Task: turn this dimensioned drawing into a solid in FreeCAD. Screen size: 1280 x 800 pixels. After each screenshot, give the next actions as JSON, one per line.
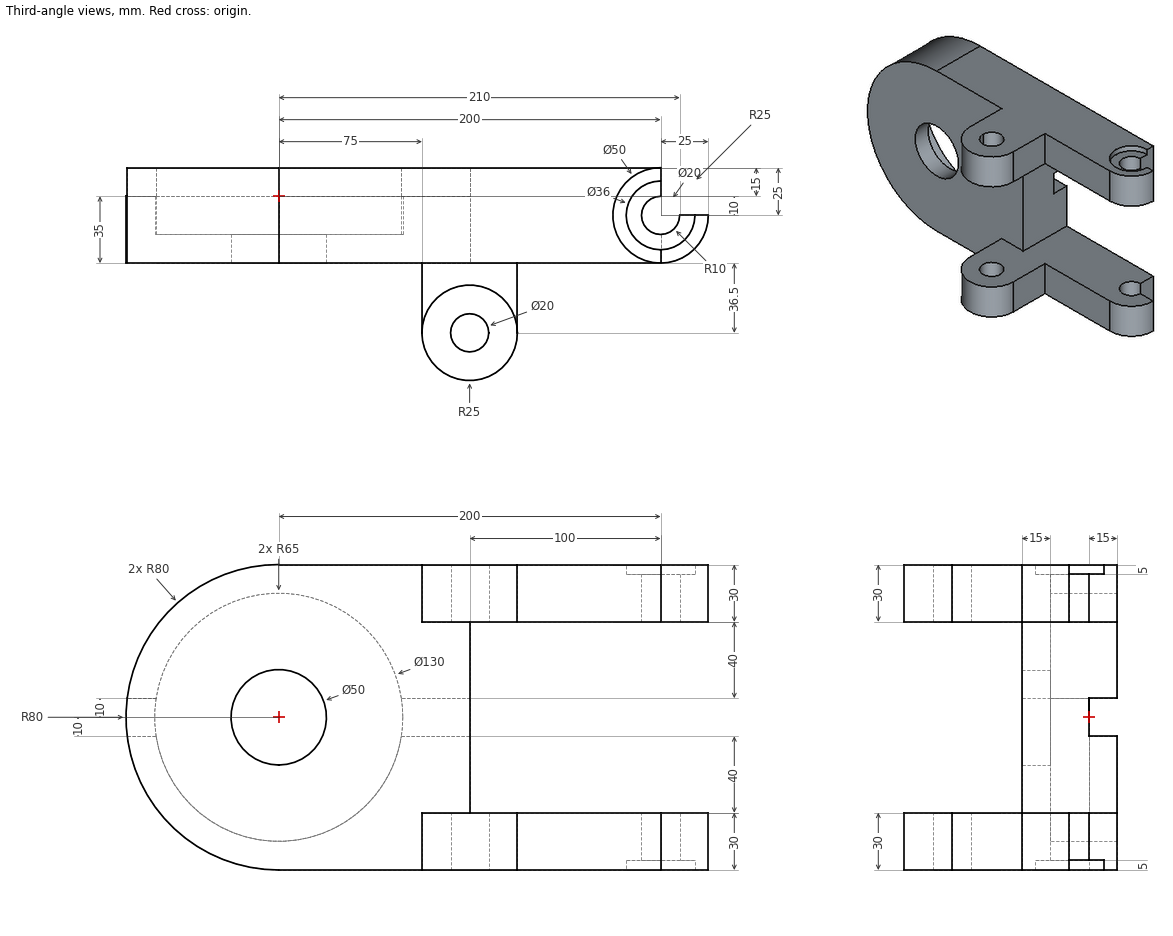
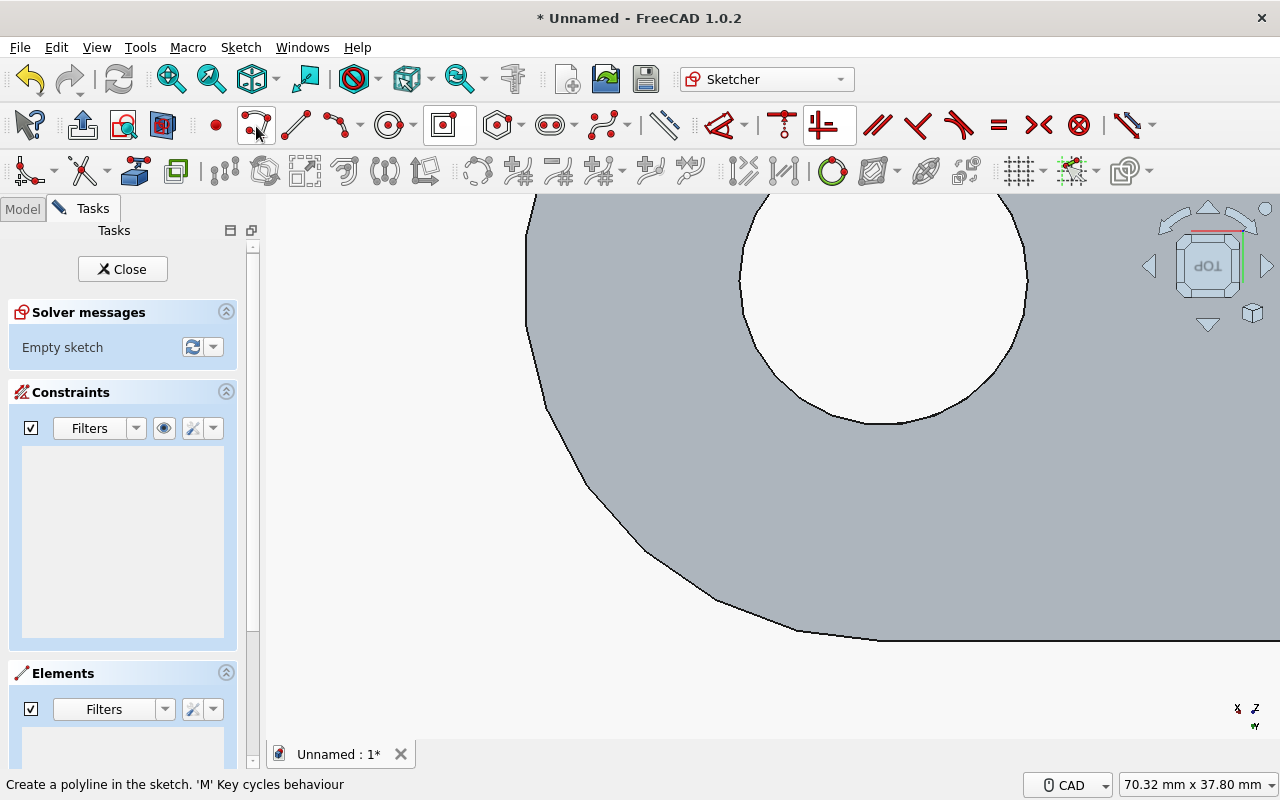
{"action": "left_click", "coordinate": [884, 641]}
{"action": "left_click", "coordinate": [884, 281]}
{"action": "left_click", "coordinate": [523, 281]}
{"action": "right_click", "coordinate": [523, 281]}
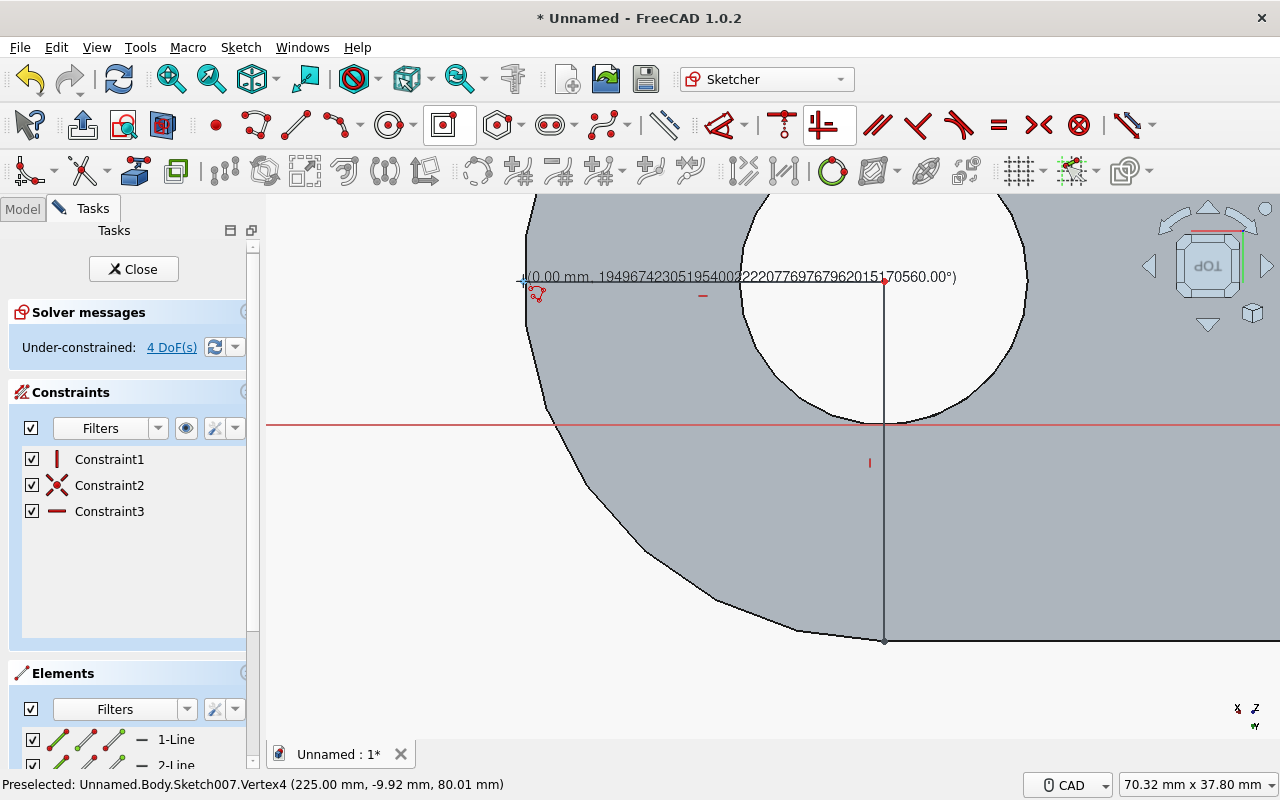
{"action": "left_click", "coordinate": [336, 126]}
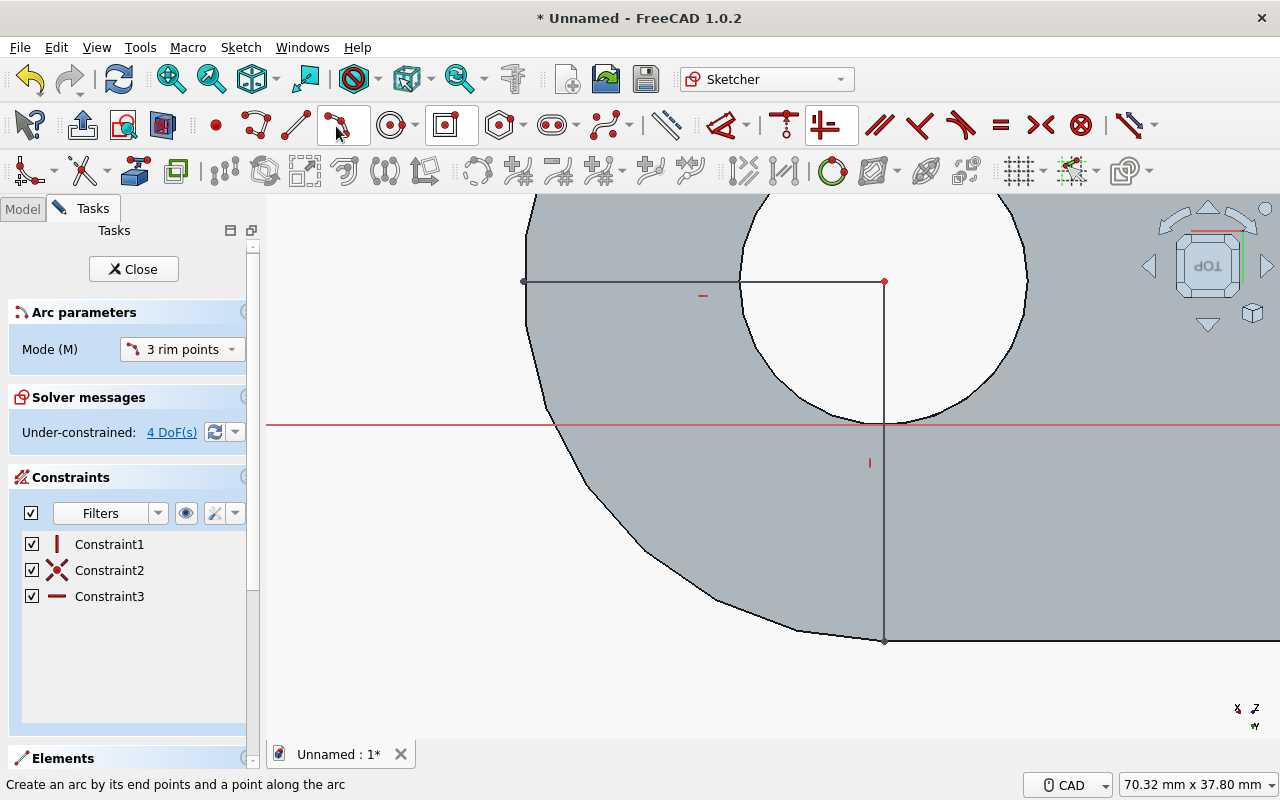
{"action": "left_click", "coordinate": [523, 282]}
{"action": "left_click", "coordinate": [884, 642]}
{"action": "left_click", "coordinate": [629, 536]}
{"action": "key", "text": "Escape"}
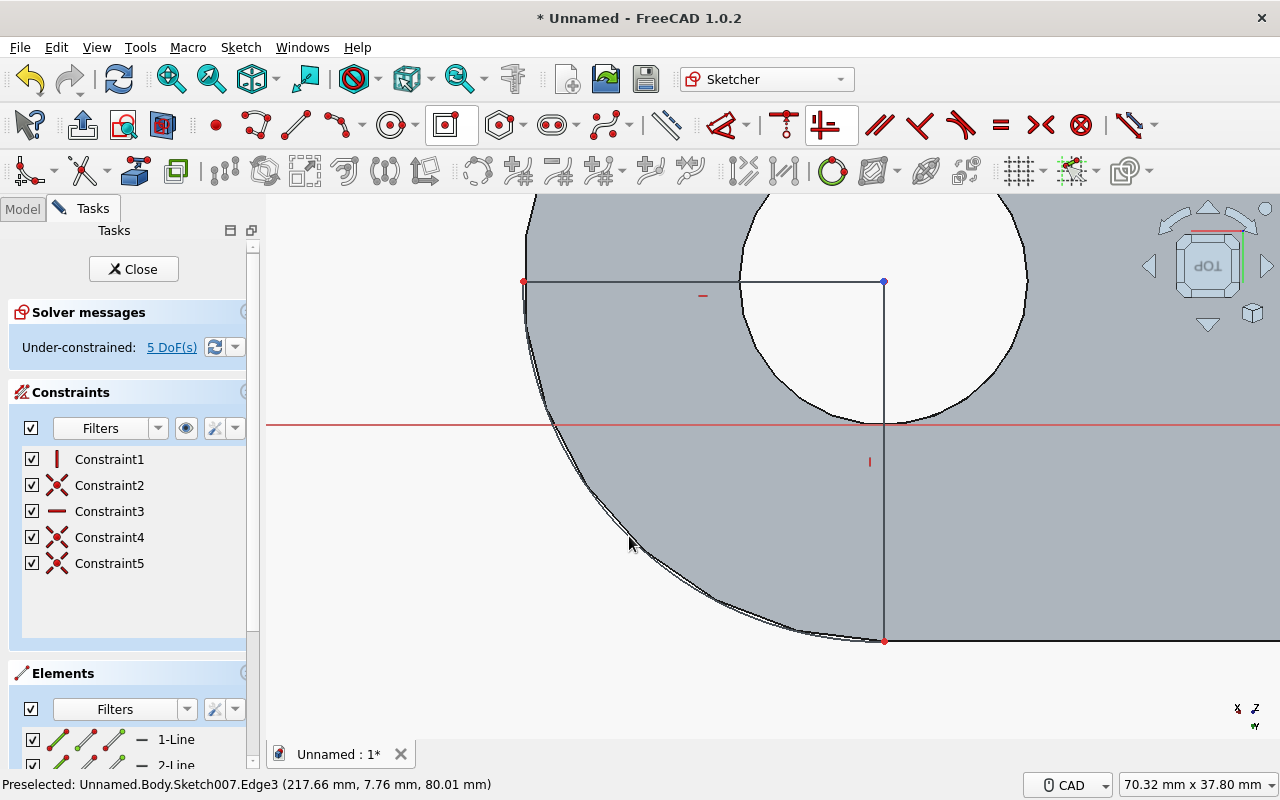
{"action": "left_click", "coordinate": [722, 126]}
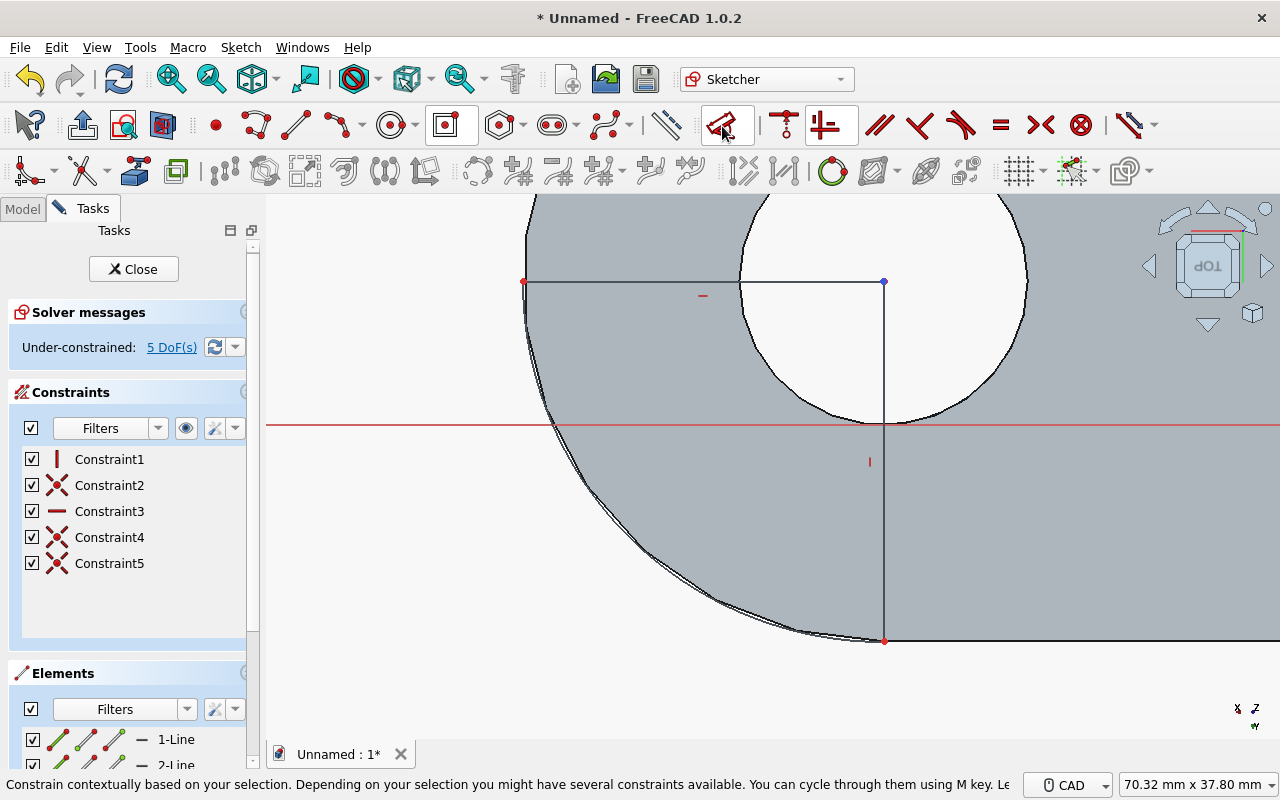
{"action": "left_click", "coordinate": [562, 446]}
{"action": "left_click", "coordinate": [534, 461]}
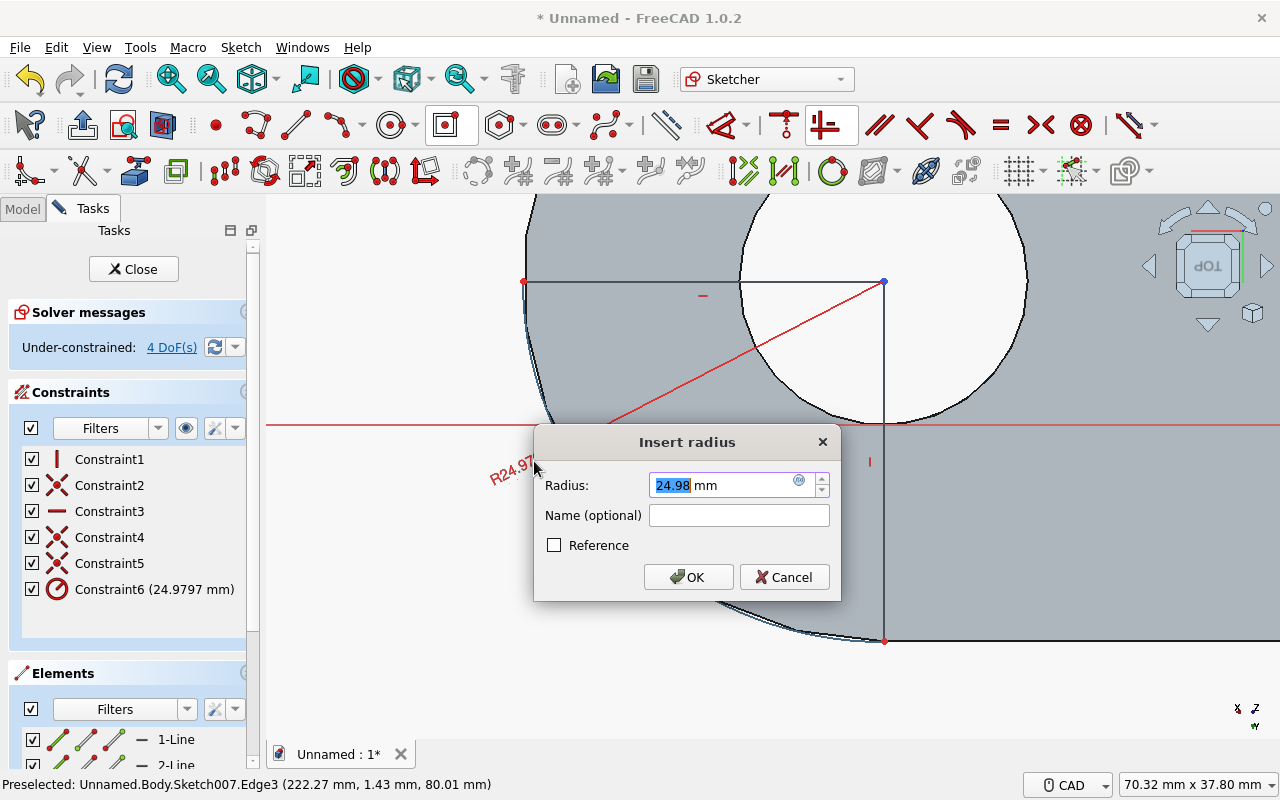
{"action": "type", "text": "25"}
{"action": "key", "text": "Return"}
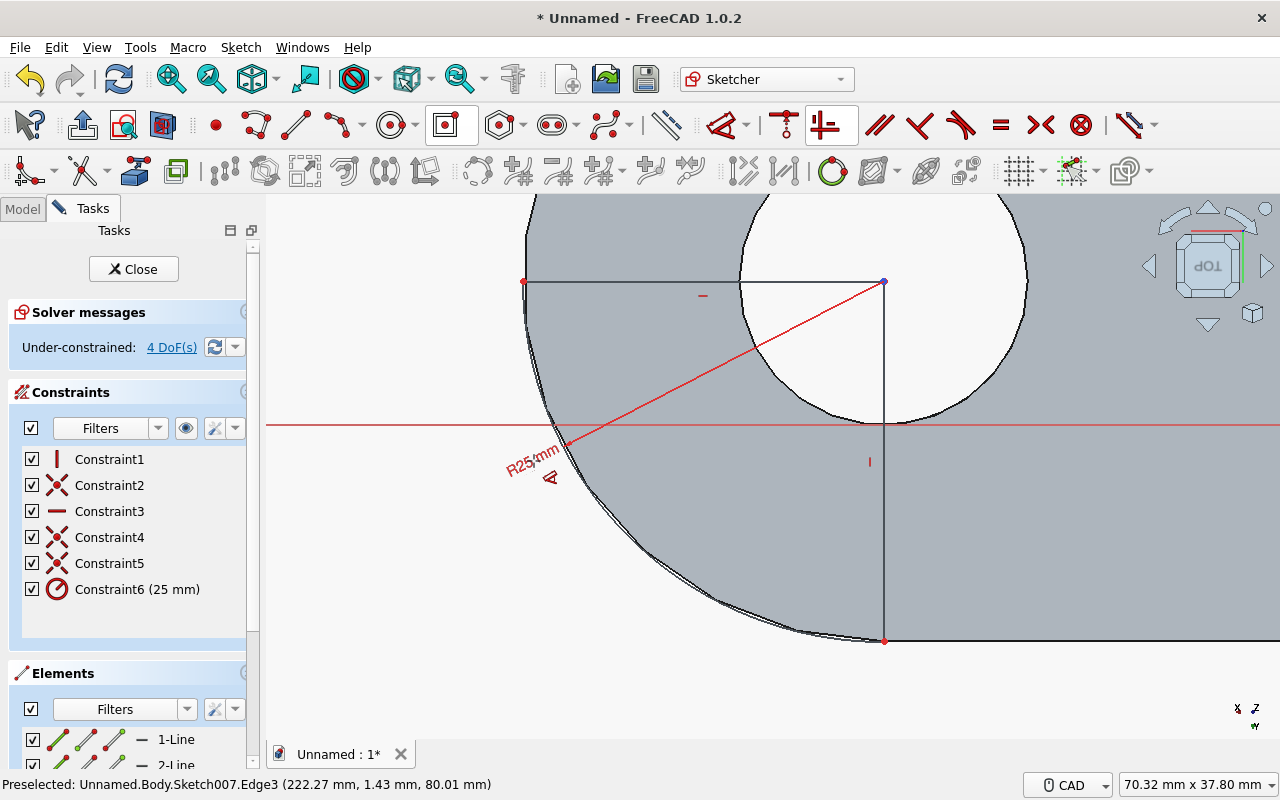
{"action": "left_click", "coordinate": [884, 534]}
{"action": "left_click", "coordinate": [918, 462]}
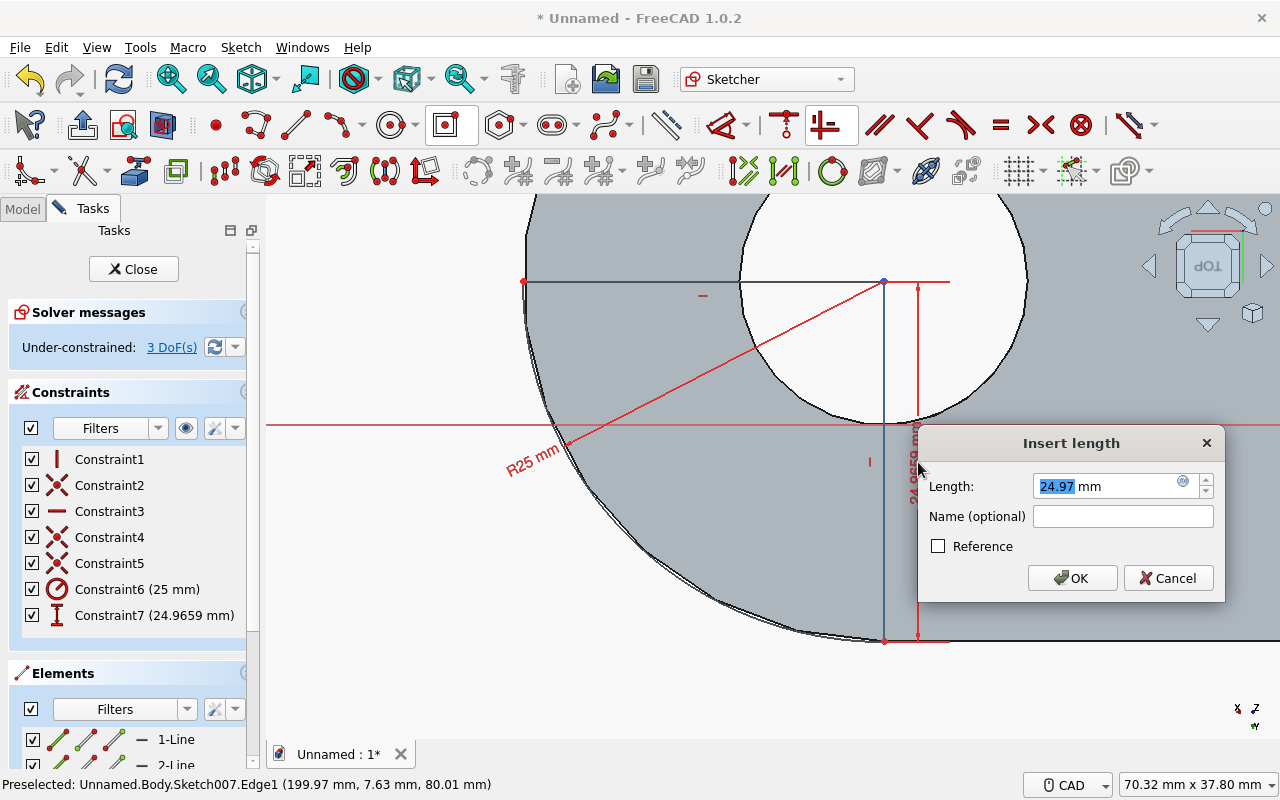
{"action": "type", "text": "25"}
{"action": "key", "text": "Return"}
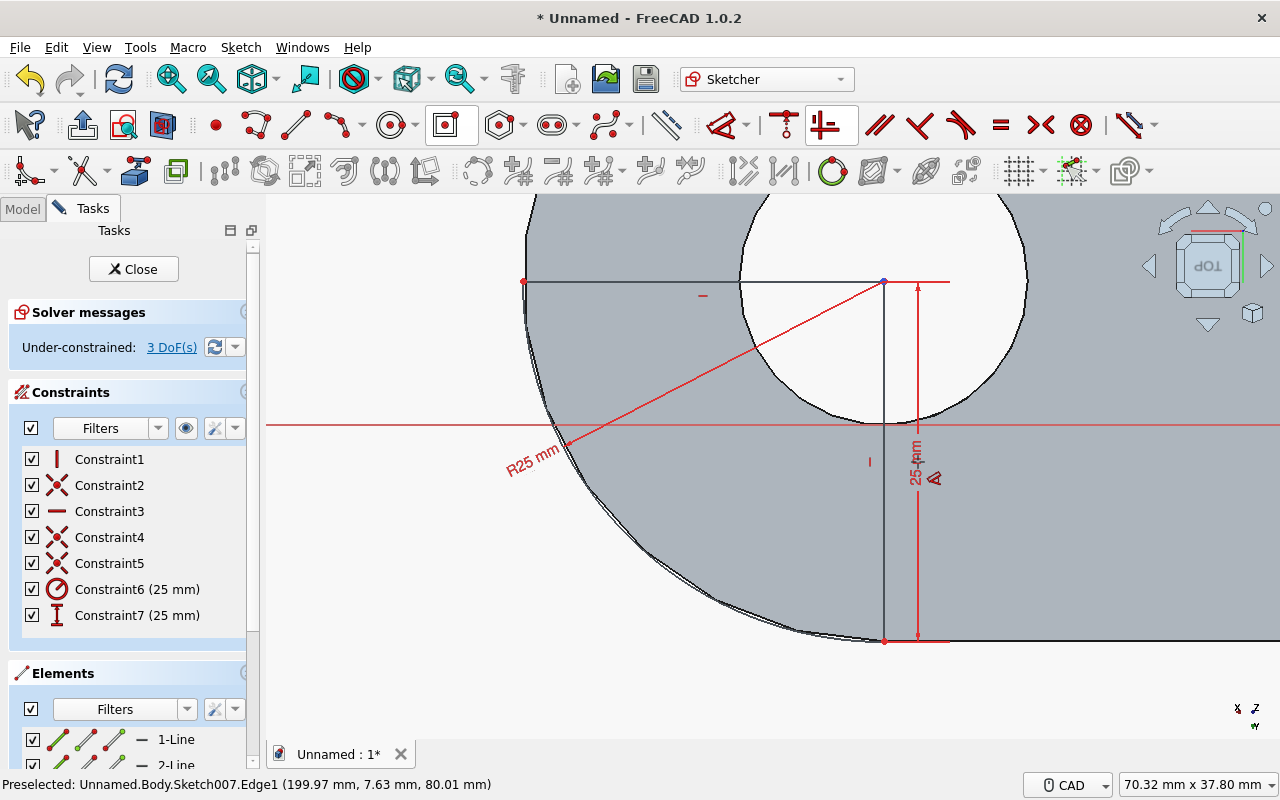
{"action": "left_click", "coordinate": [776, 282]}
{"action": "left_click", "coordinate": [704, 248]}